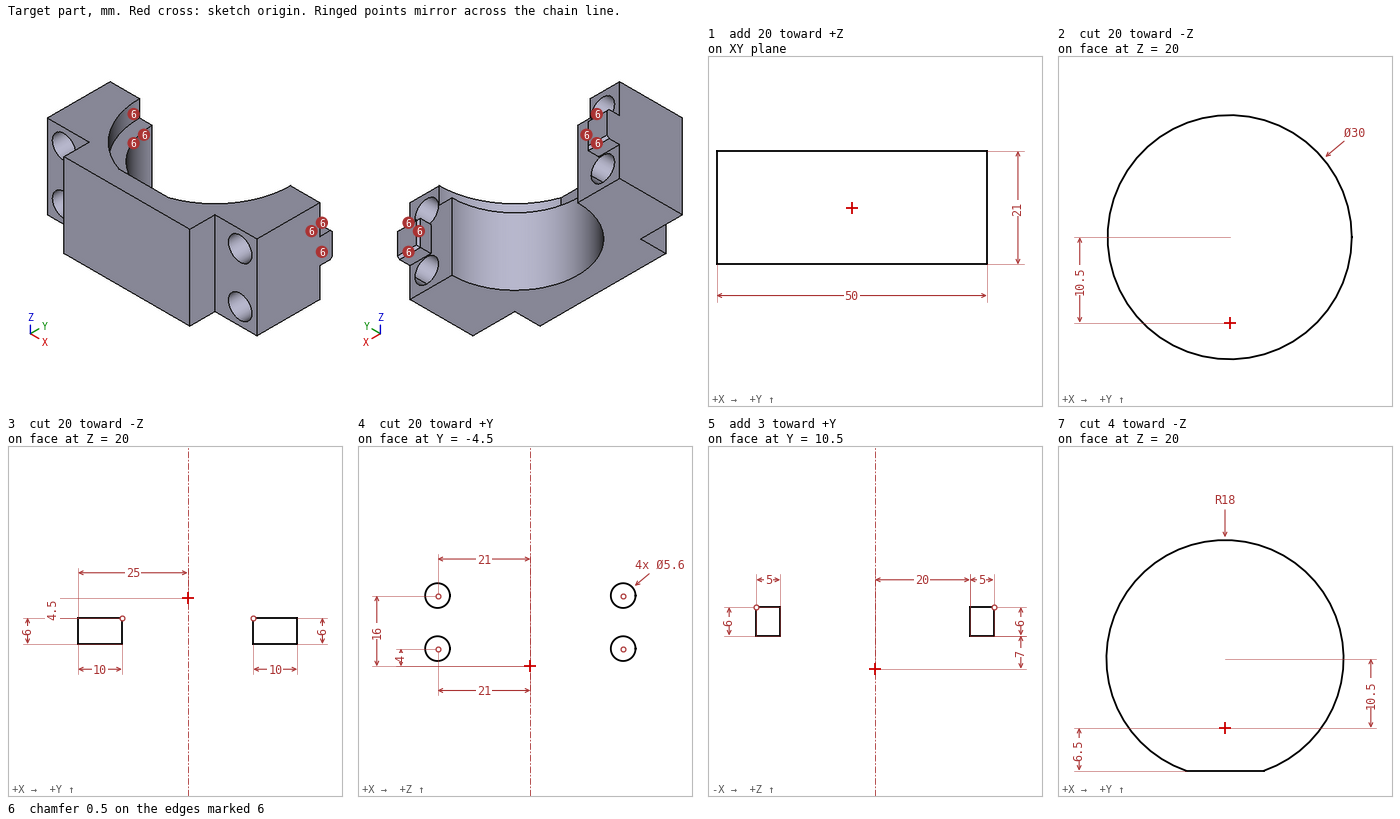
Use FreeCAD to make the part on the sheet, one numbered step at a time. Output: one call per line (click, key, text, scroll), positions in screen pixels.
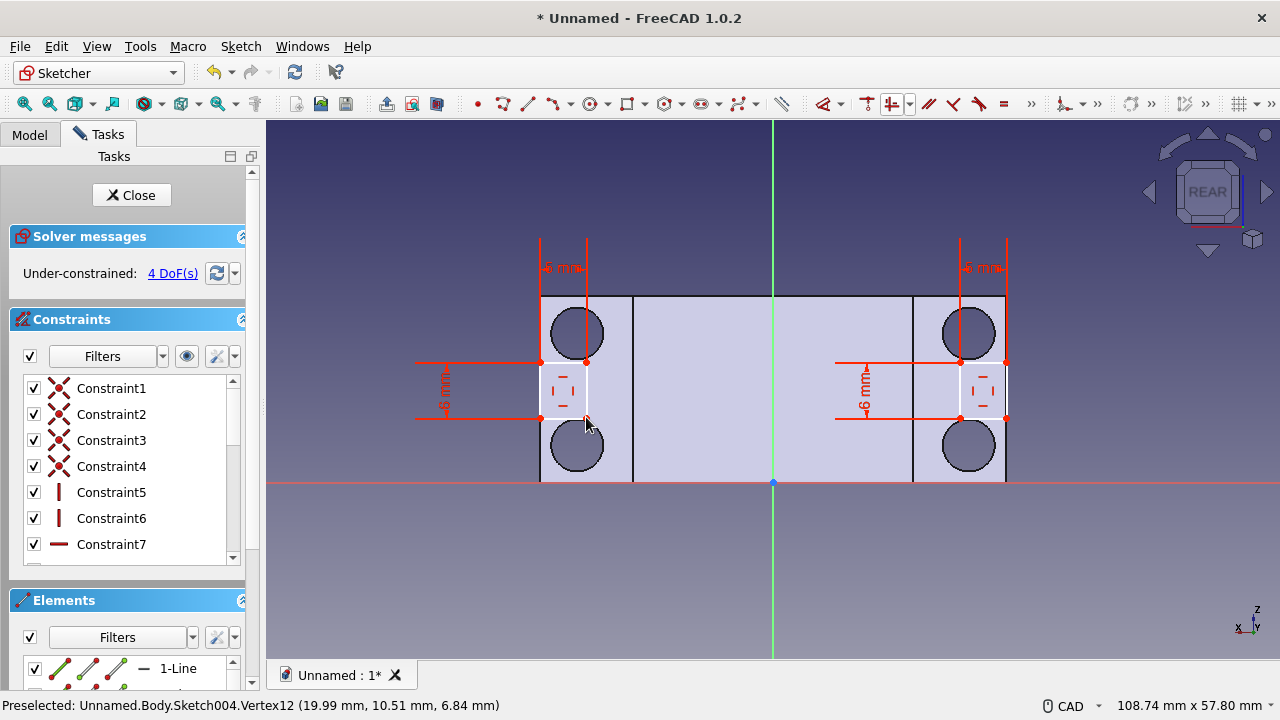
click(1007, 363)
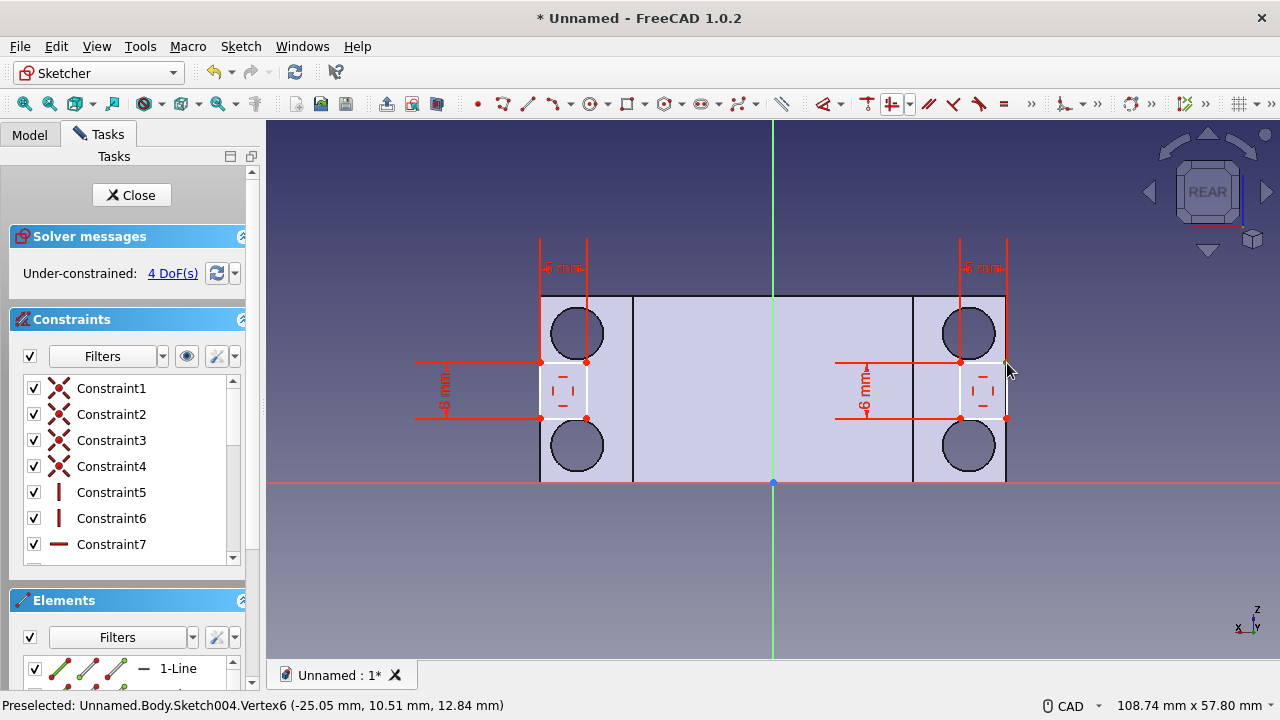
click(540, 363)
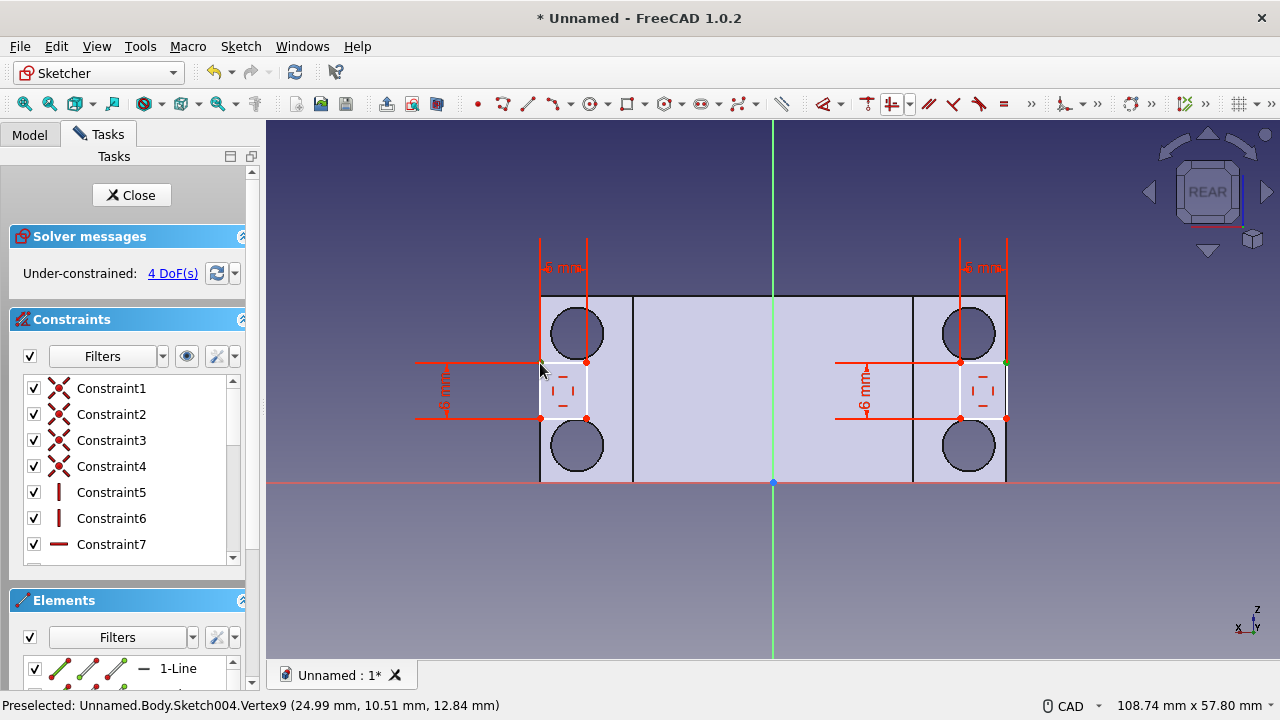
click(773, 596)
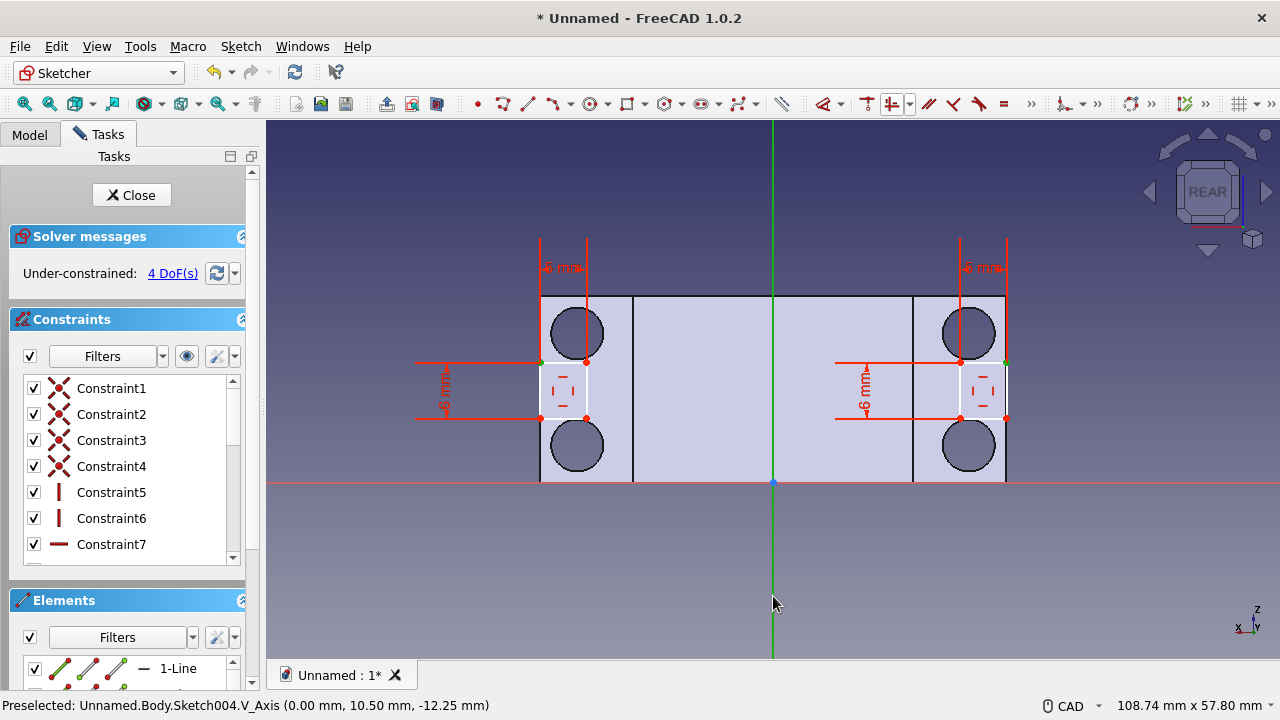
key(s)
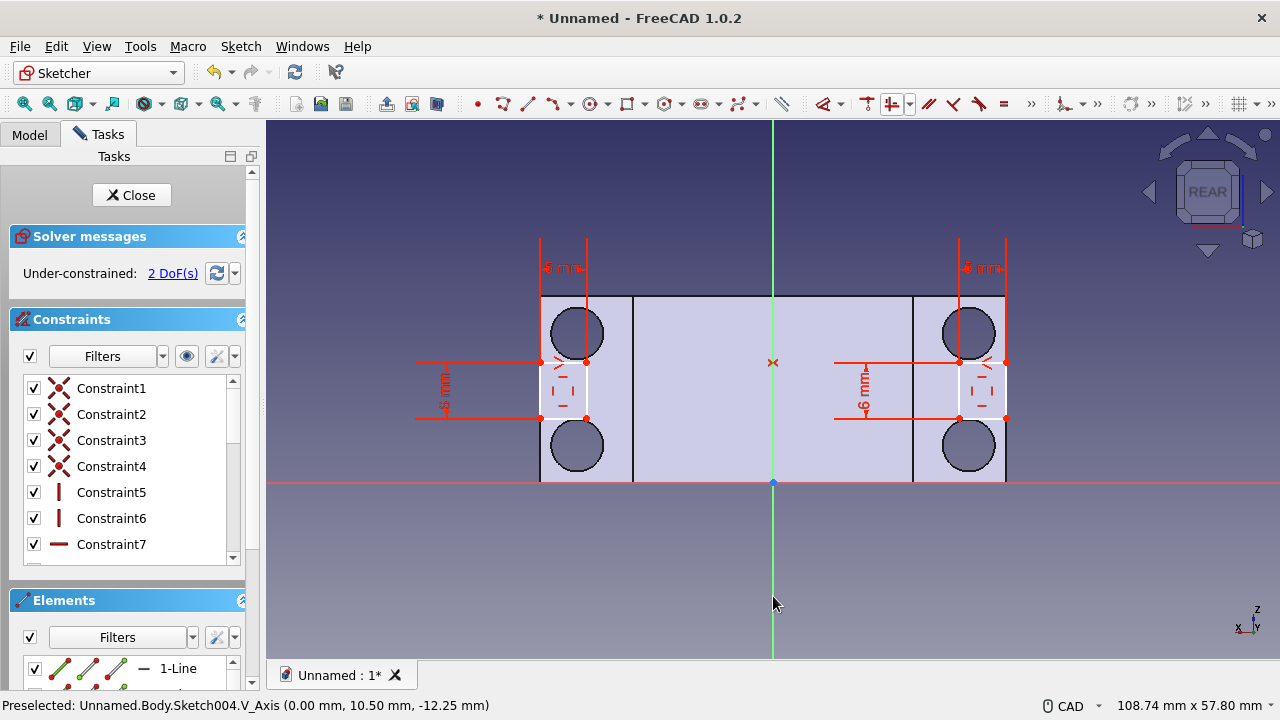
click(822, 104)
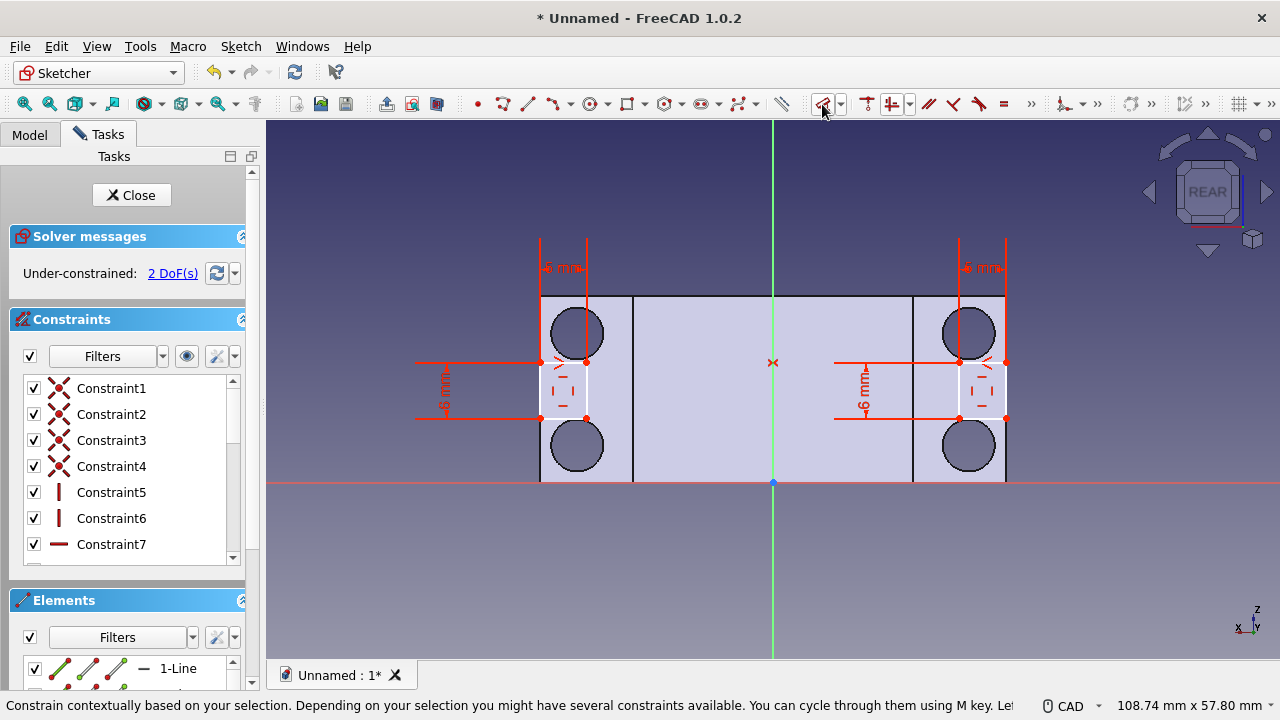
click(959, 419)
click(993, 451)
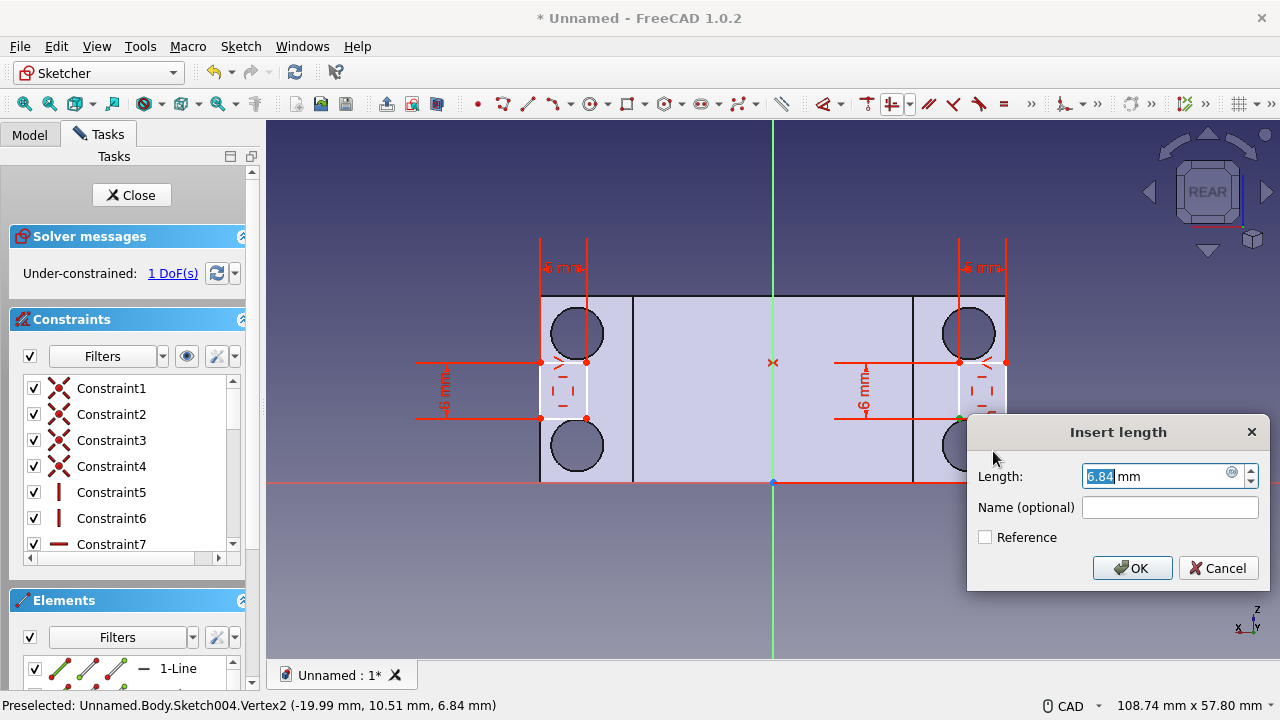
text(7)
key(Return)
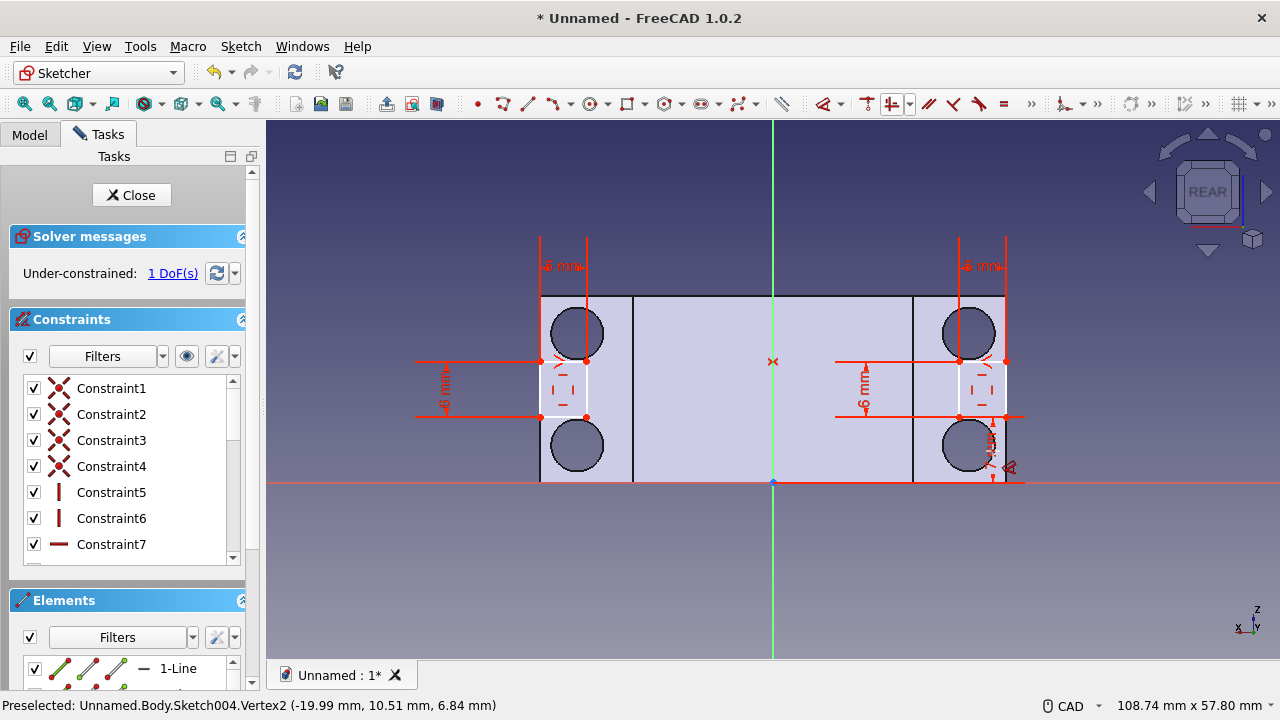
click(959, 362)
click(866, 517)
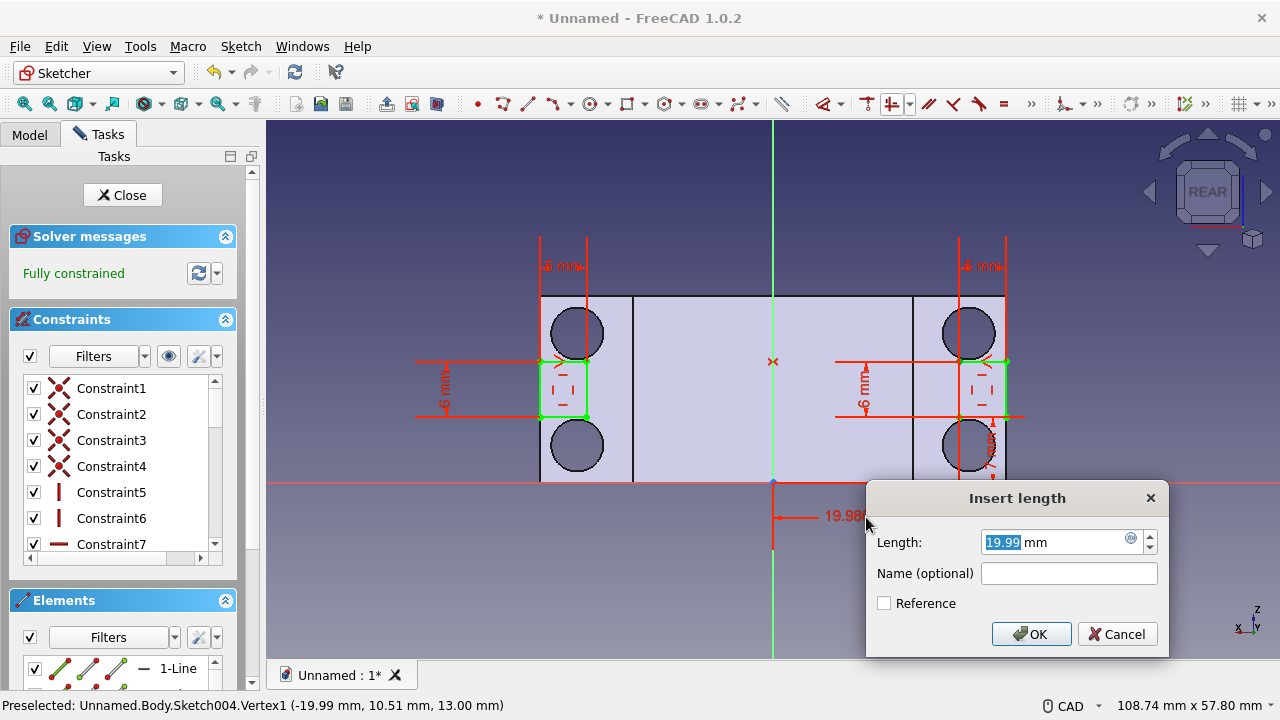
text(20)
key(Return)
key(Escape)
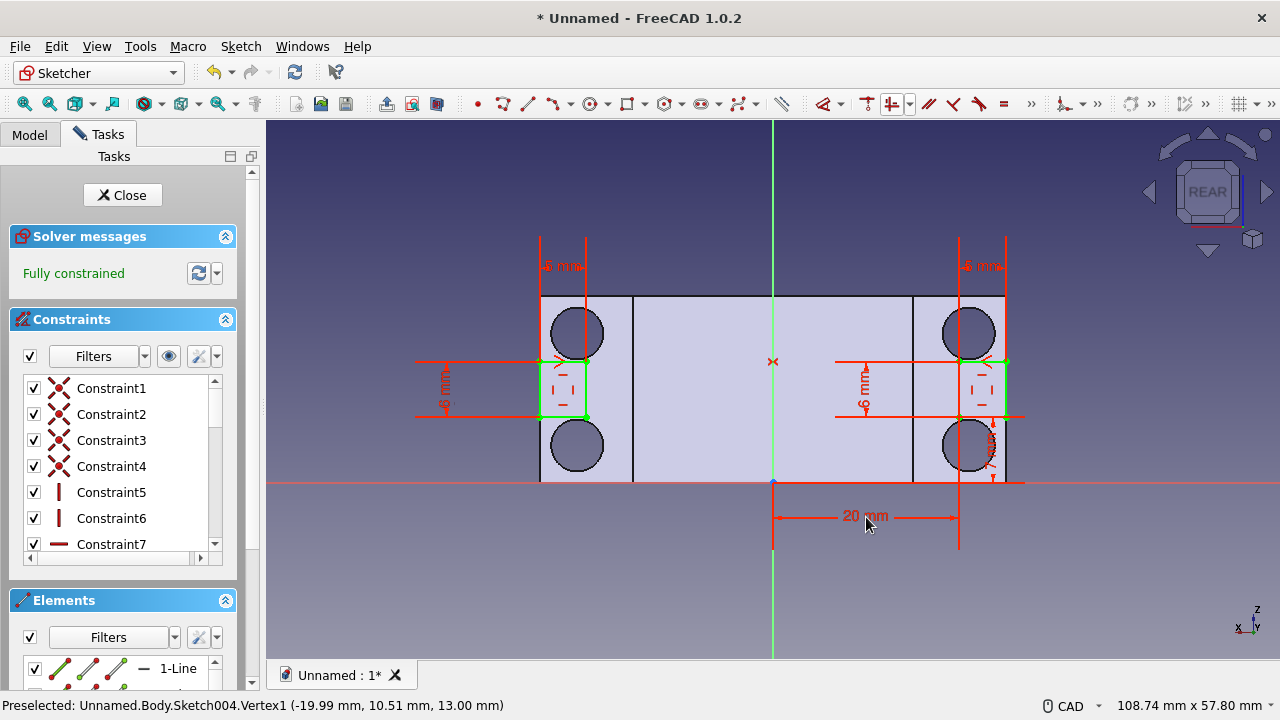
click(123, 195)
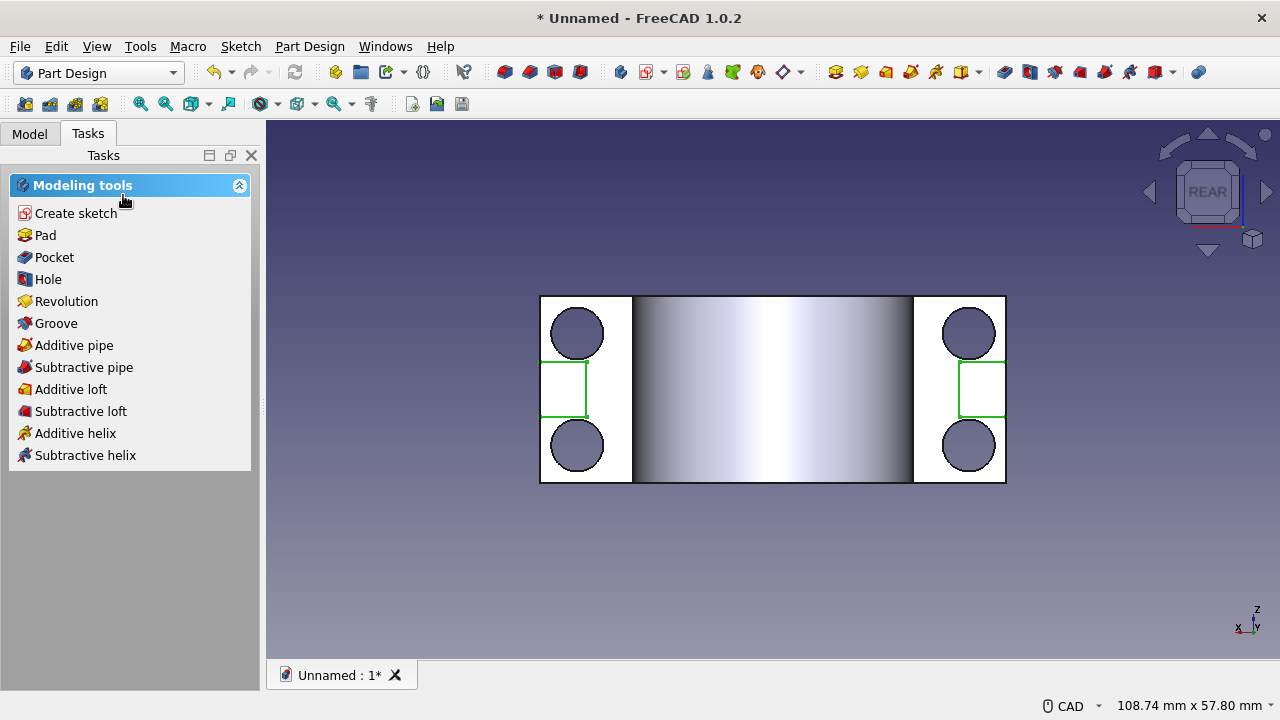
click(836, 72)